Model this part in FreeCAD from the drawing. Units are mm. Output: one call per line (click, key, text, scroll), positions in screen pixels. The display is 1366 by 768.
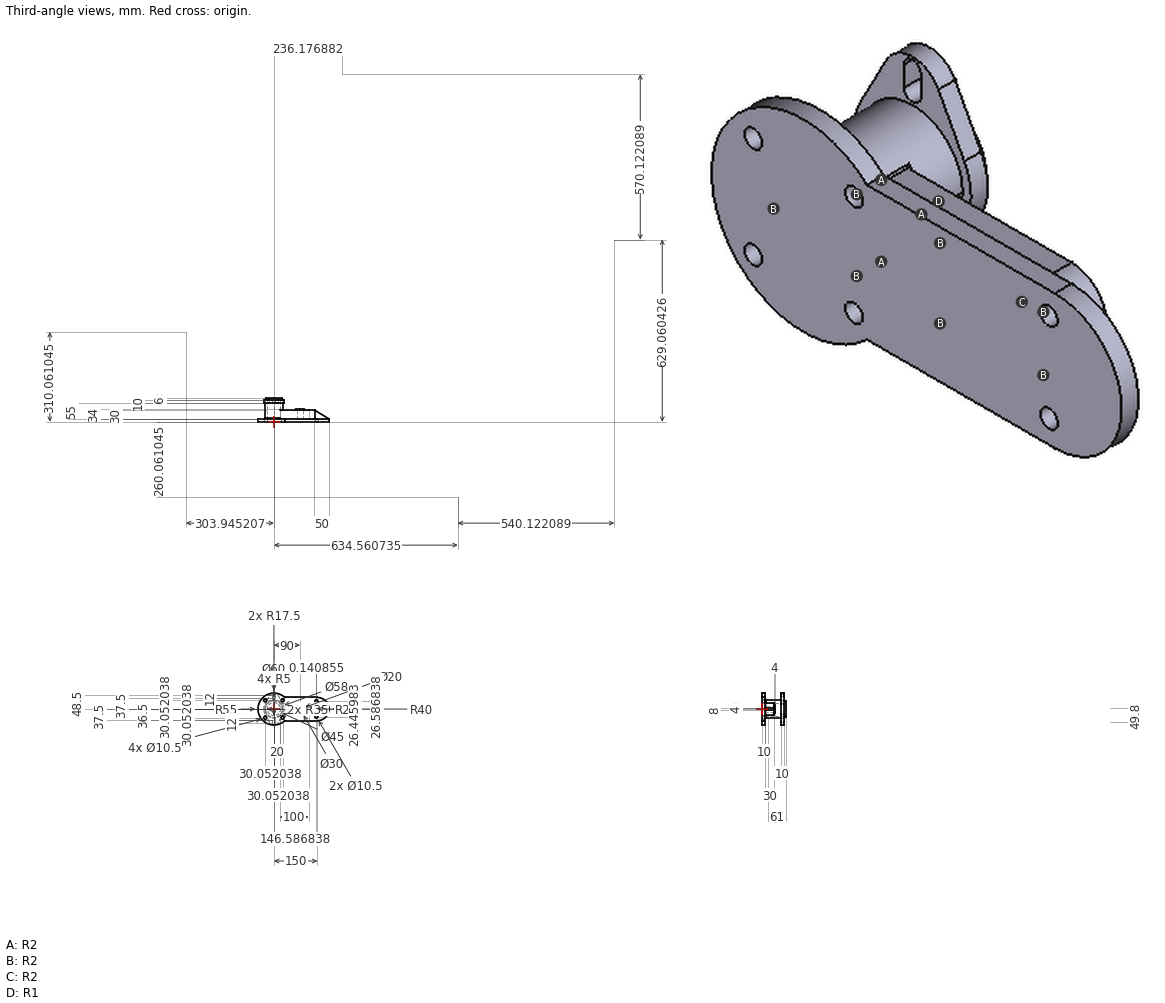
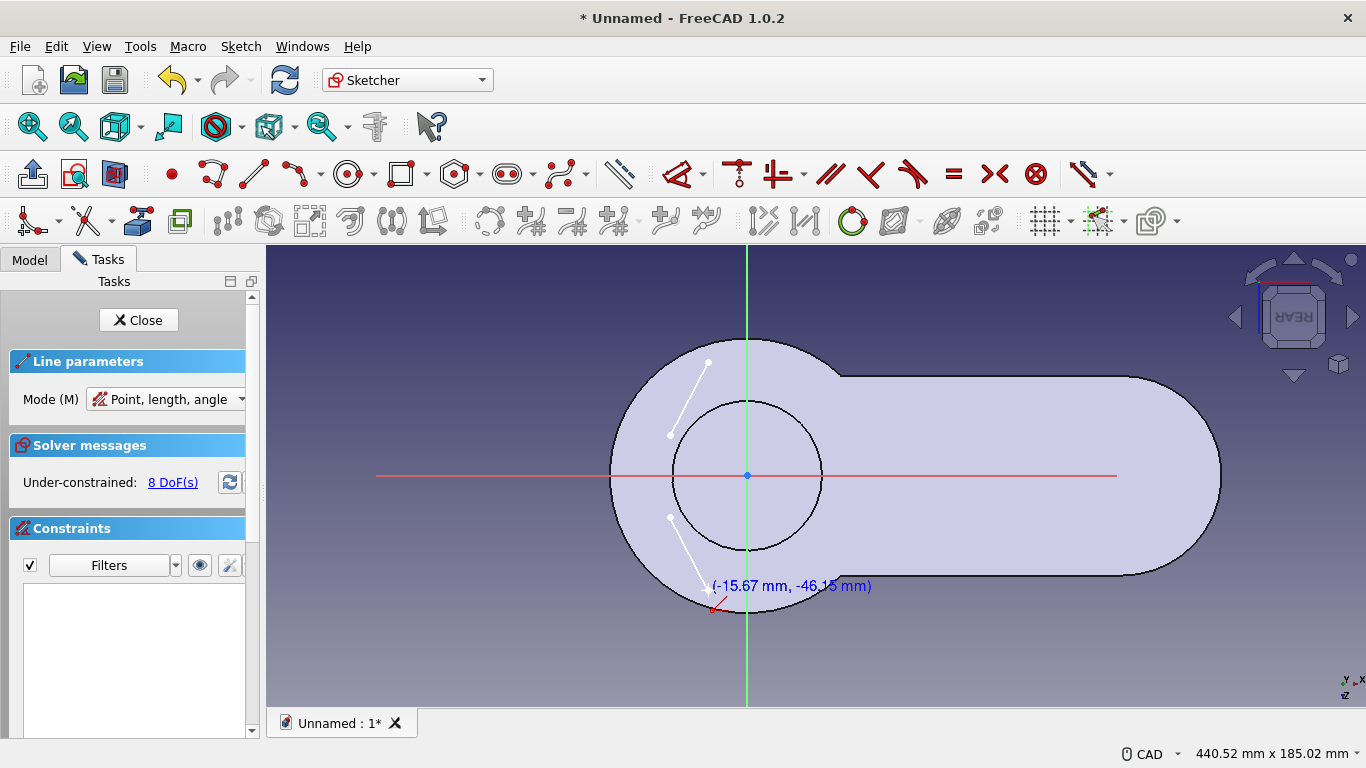
click(786, 590)
click(824, 517)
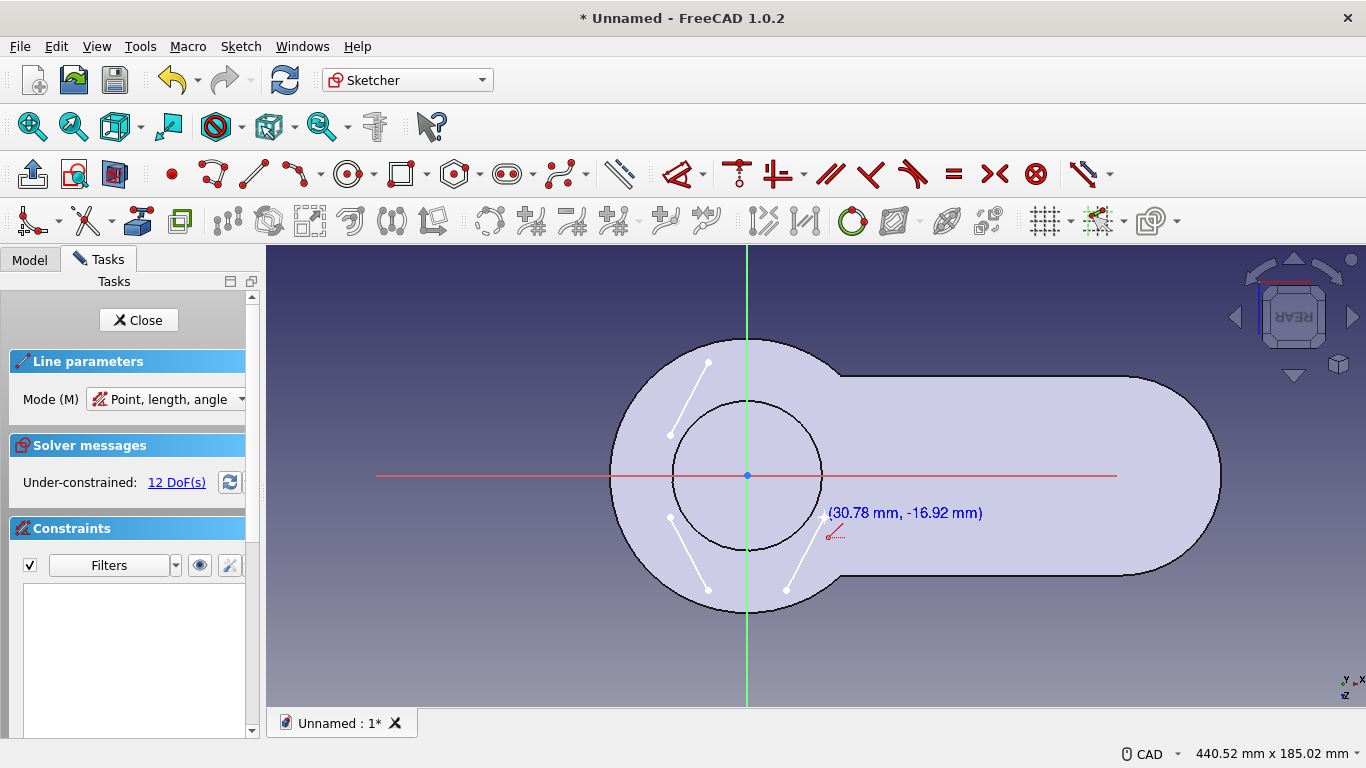
click(824, 435)
click(786, 362)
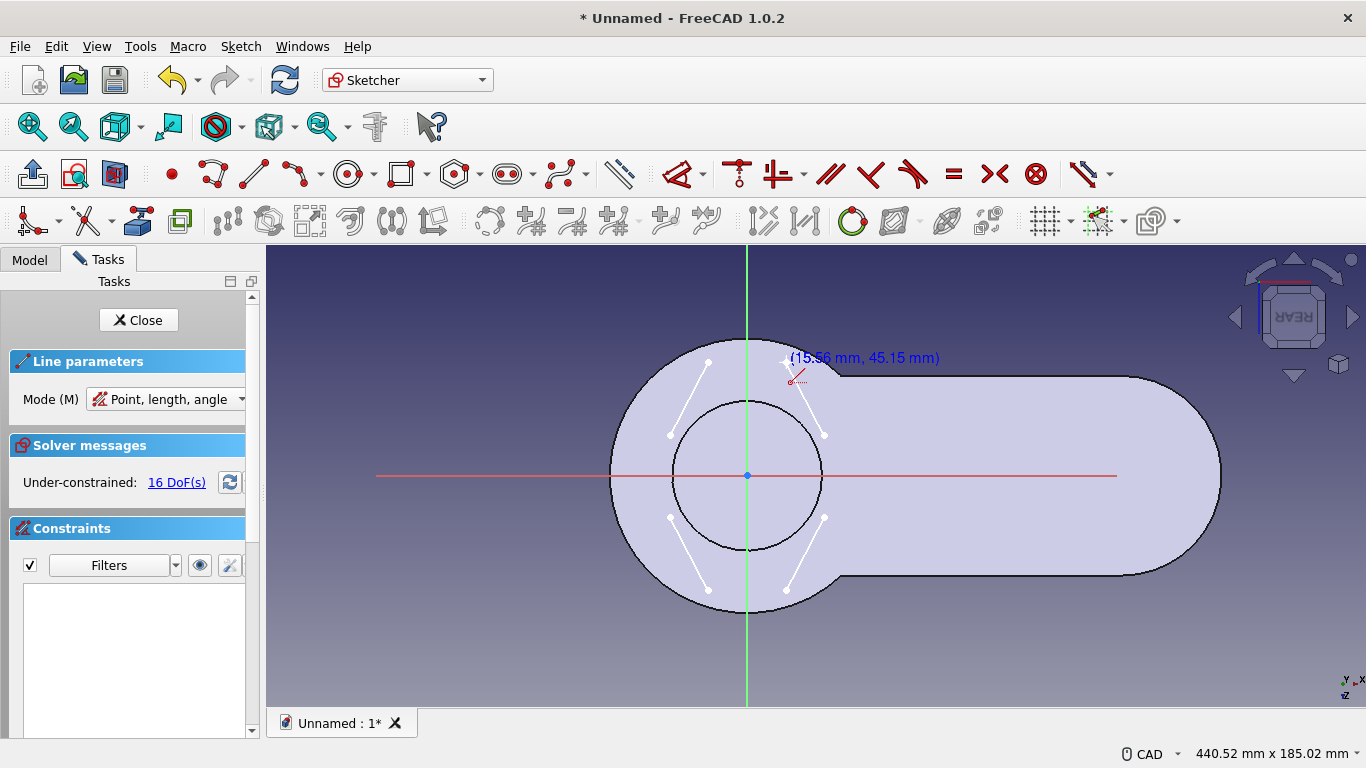
key(g)
key(3)
key(a)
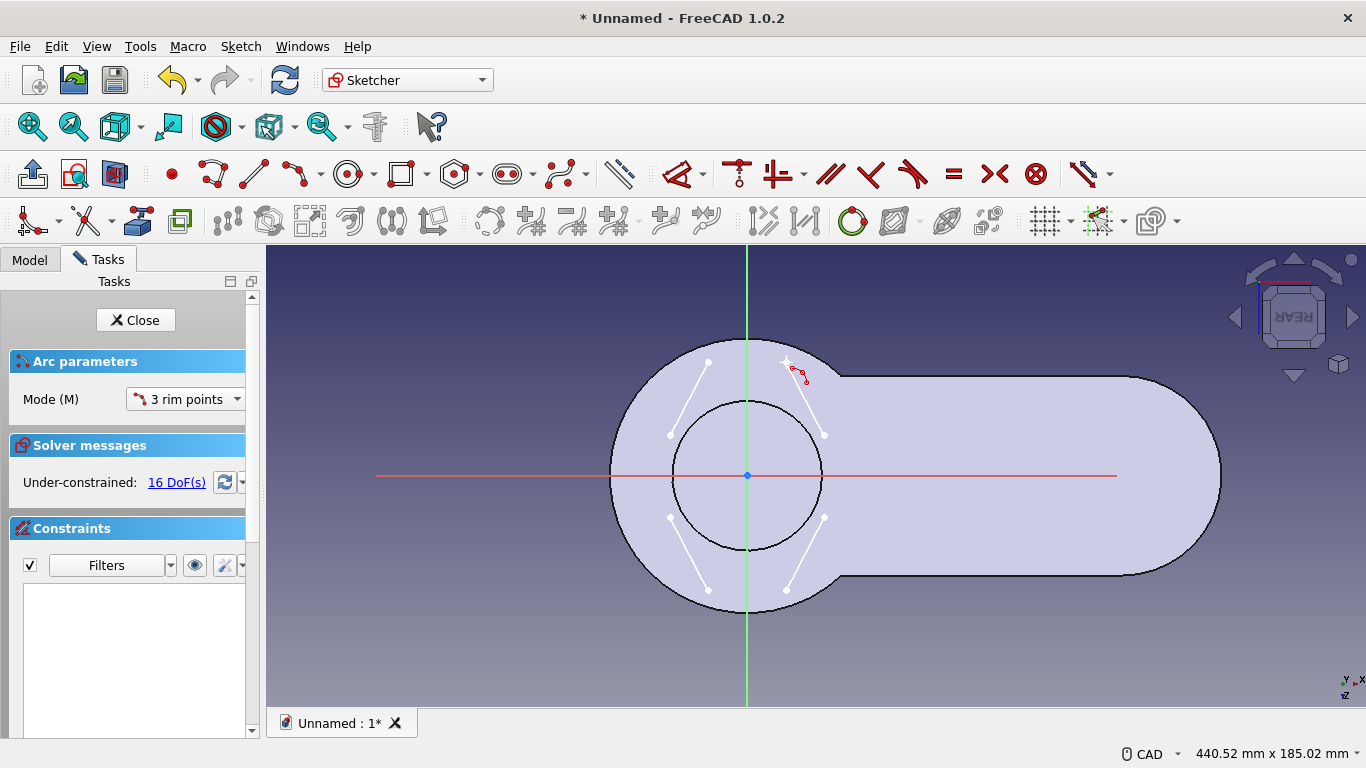
click(670, 436)
click(670, 518)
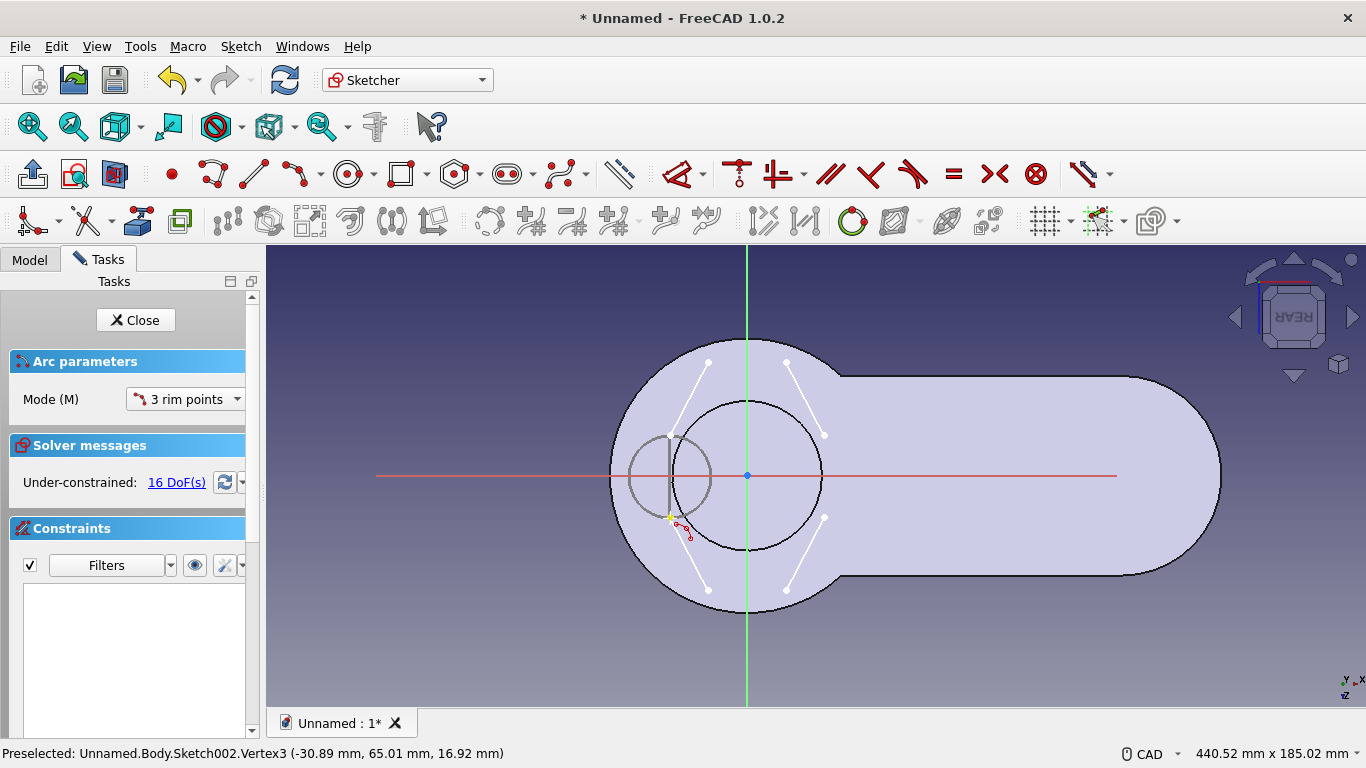
scroll(660, 467, up, 4)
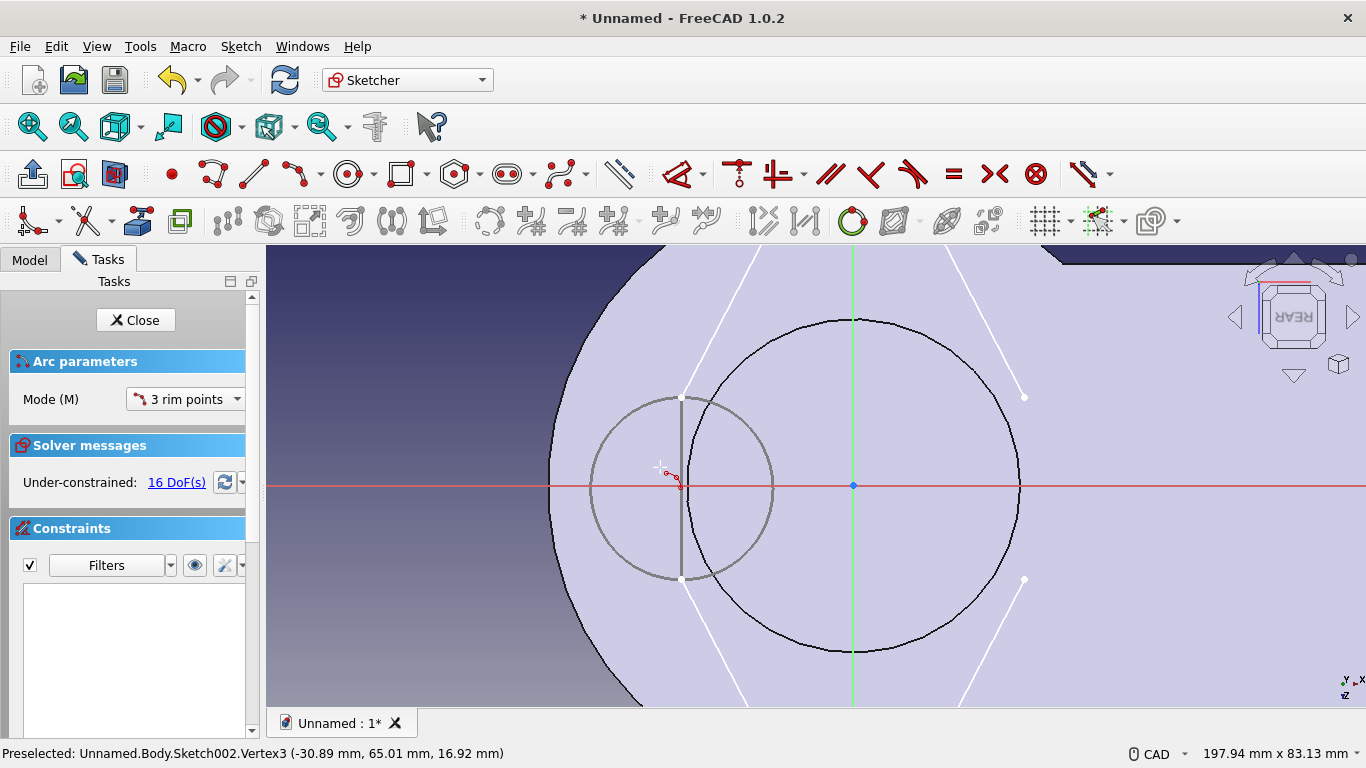
click(660, 467)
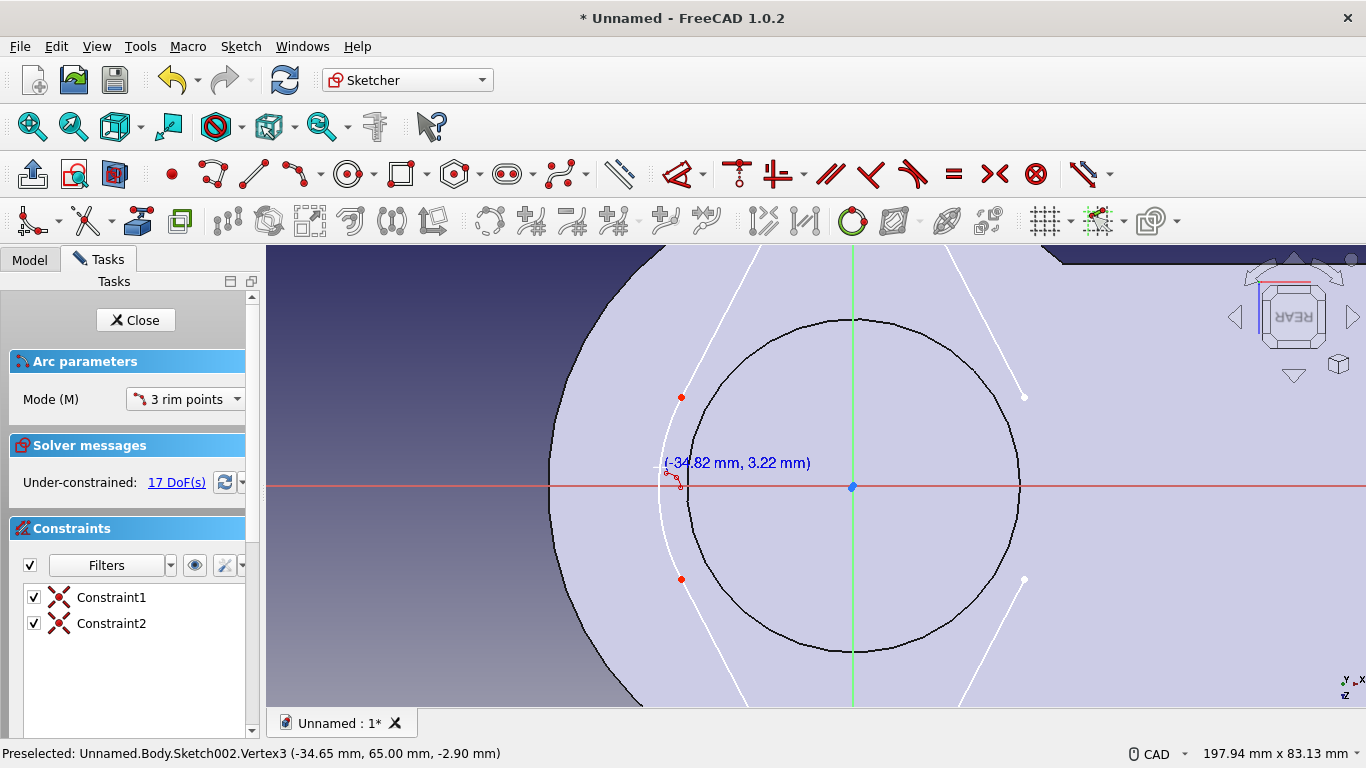
scroll(661, 468, down, 4)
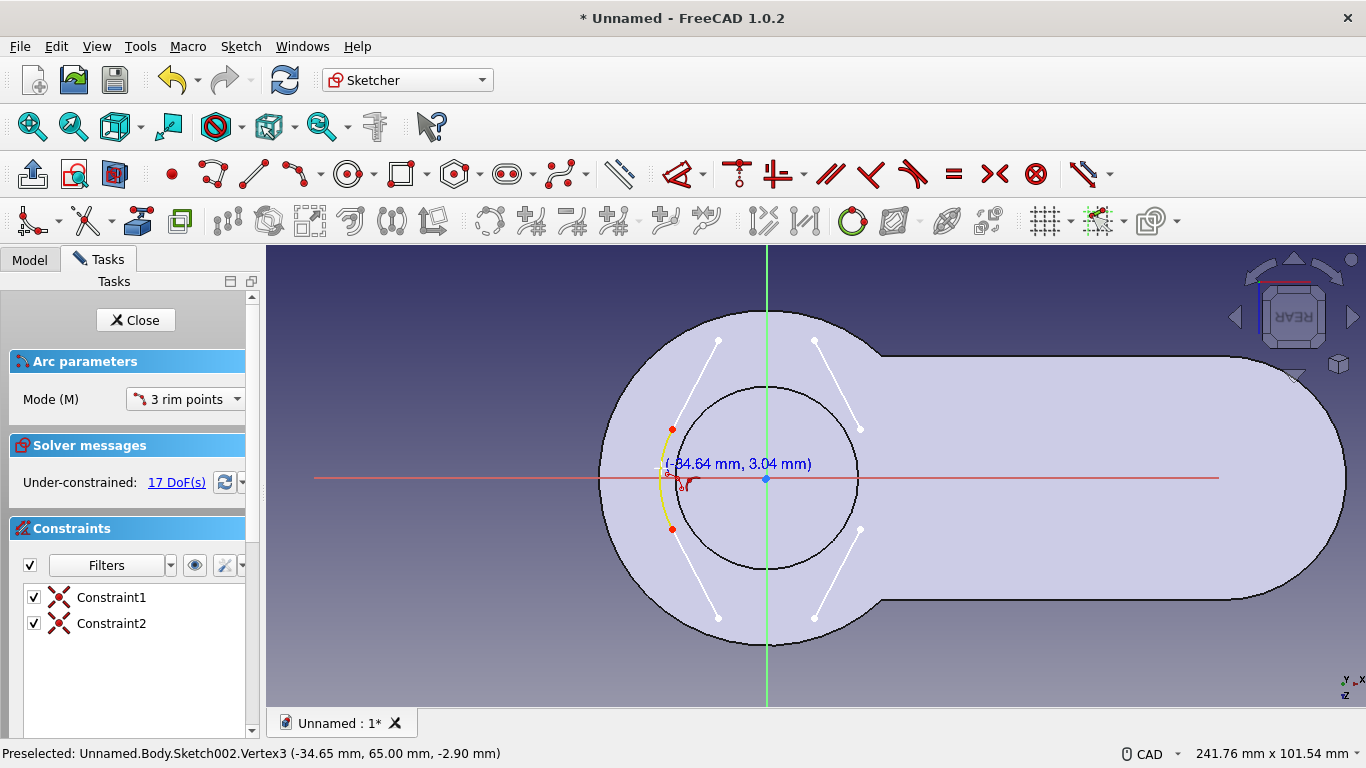
click(709, 592)
click(787, 592)
click(729, 610)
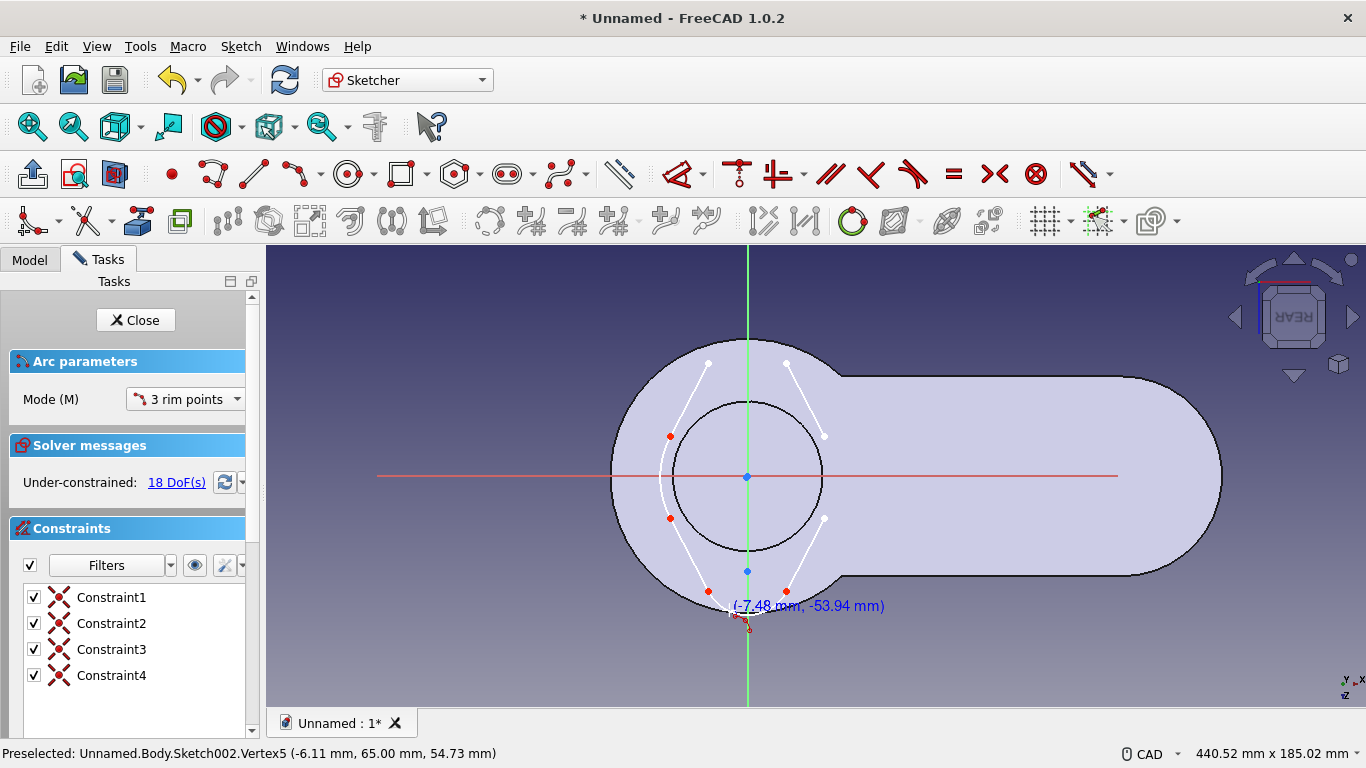
click(825, 519)
click(825, 437)